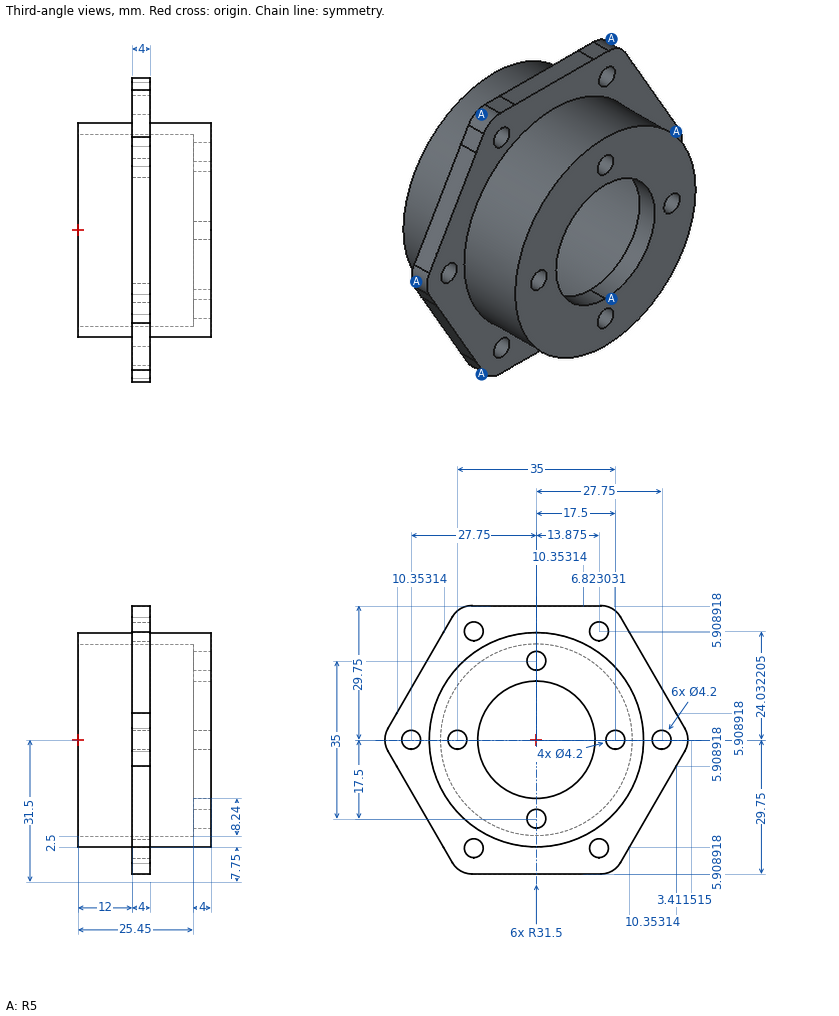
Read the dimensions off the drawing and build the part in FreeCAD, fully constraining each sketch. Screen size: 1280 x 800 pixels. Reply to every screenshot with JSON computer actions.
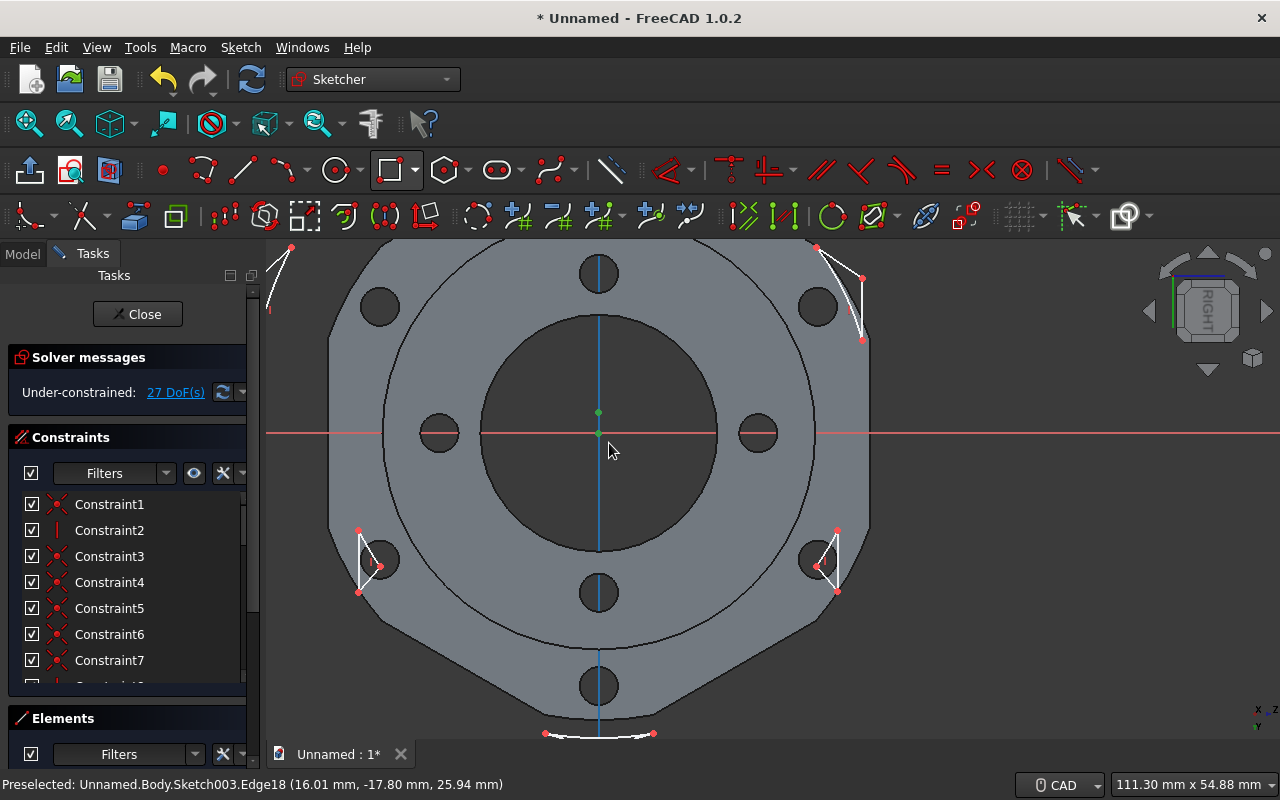
{"action": "key", "text": "c"}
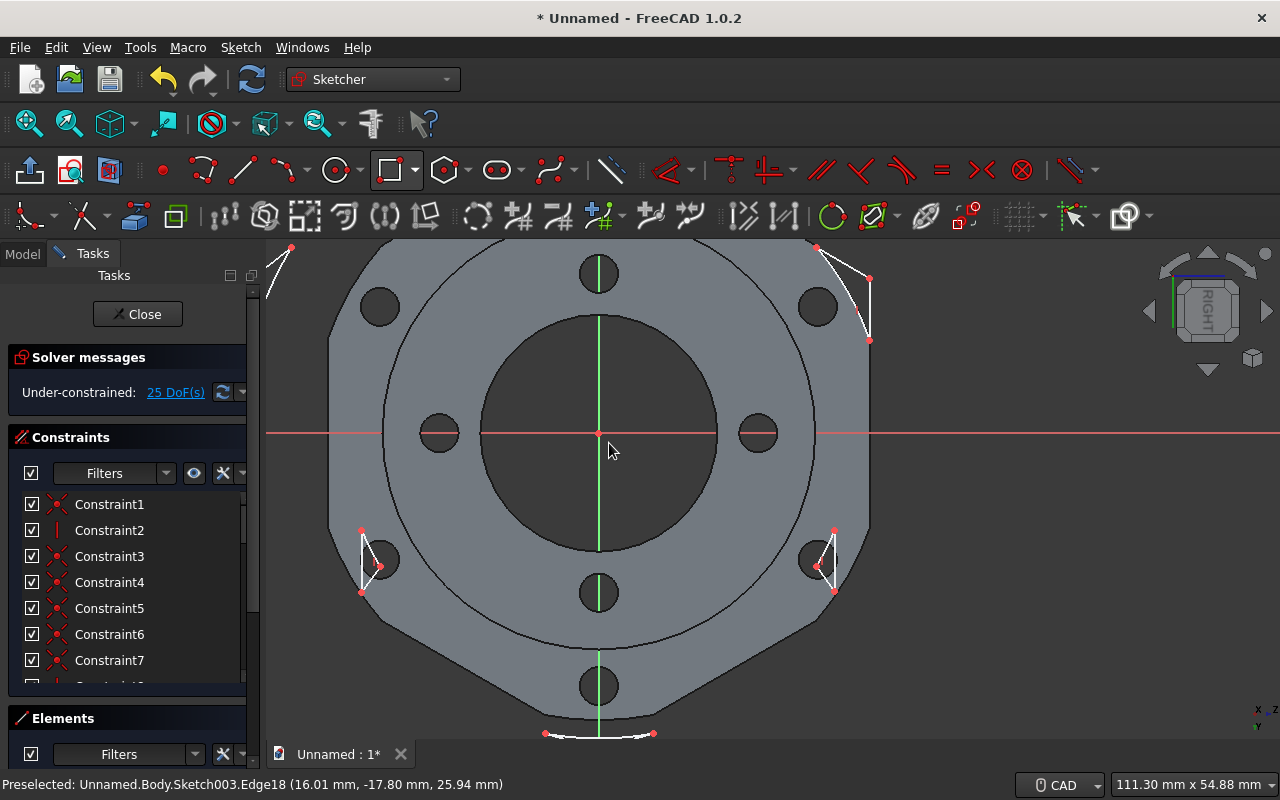
{"action": "left_click", "coordinate": [826, 548]}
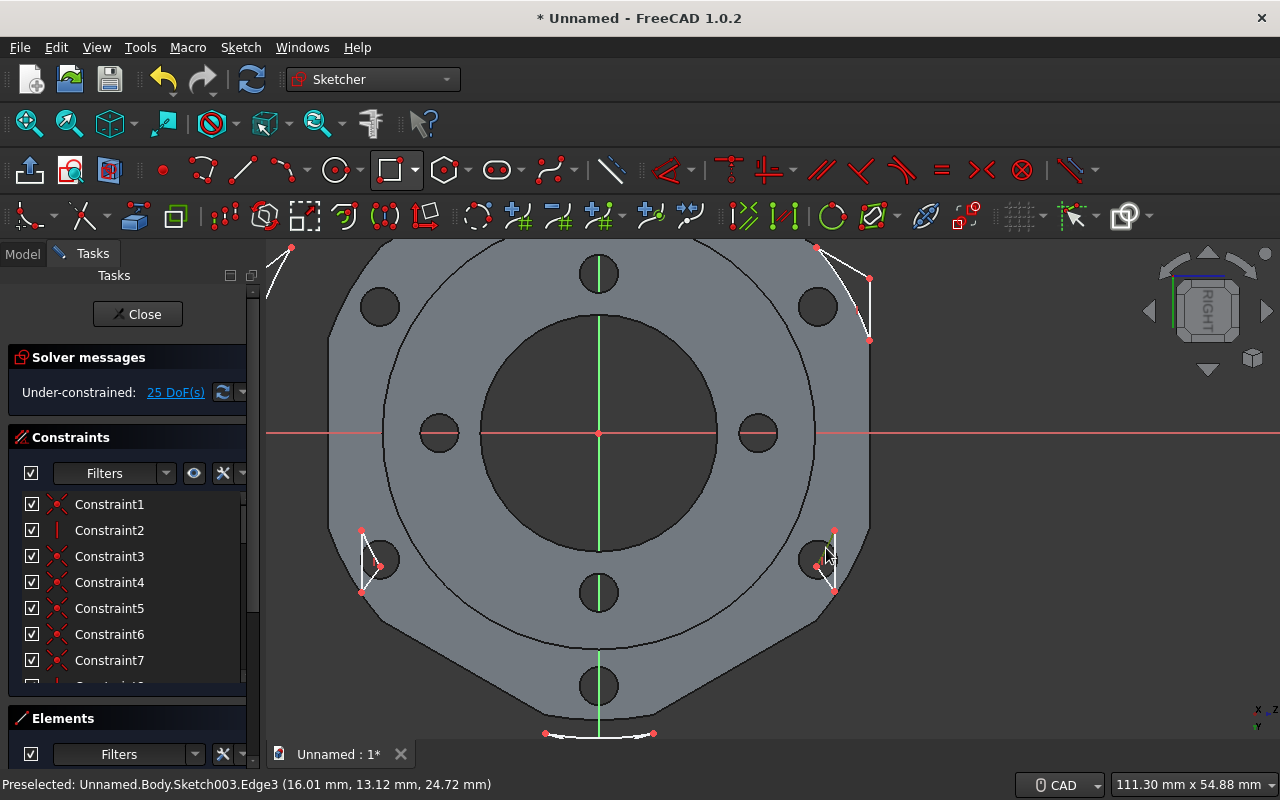
{"action": "scroll", "coordinate": [833, 557], "scroll_direction": "down", "scroll_amount": 3}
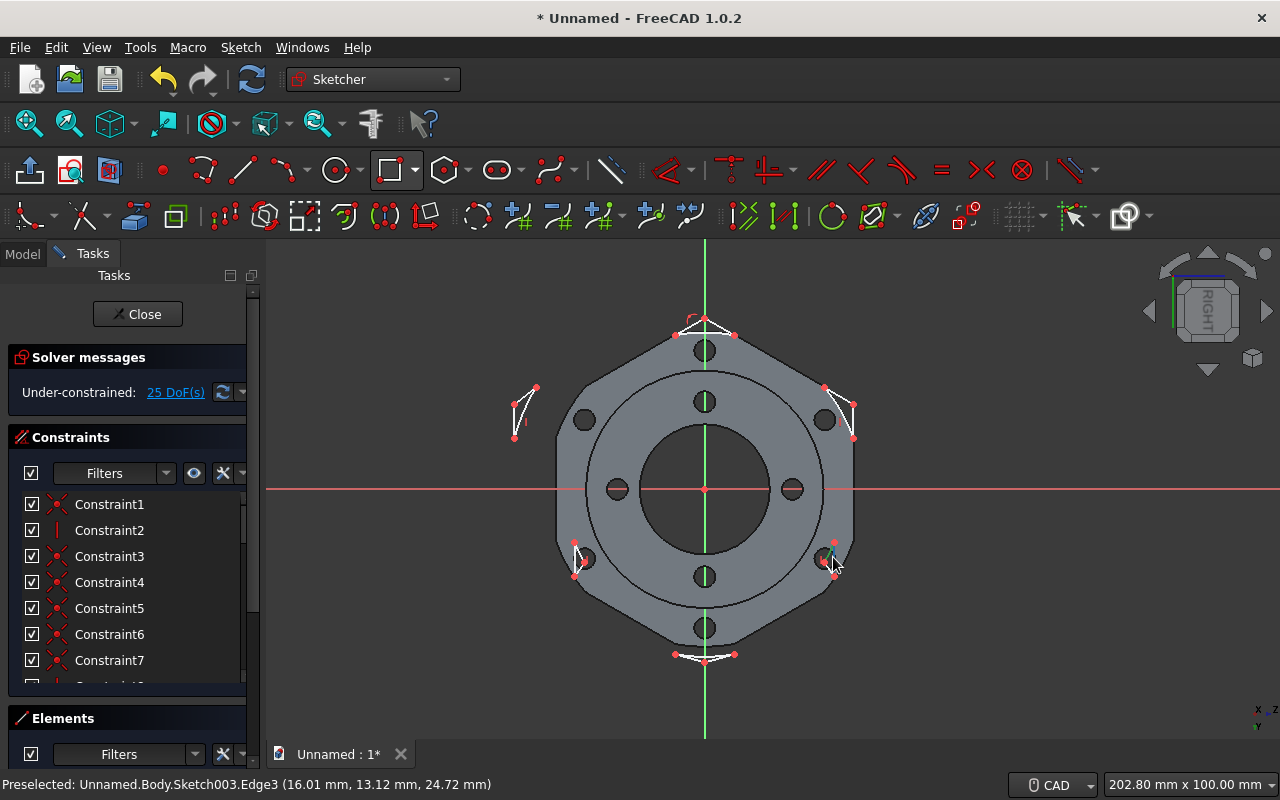
{"action": "scroll", "coordinate": [705, 657], "scroll_direction": "up", "scroll_amount": 5}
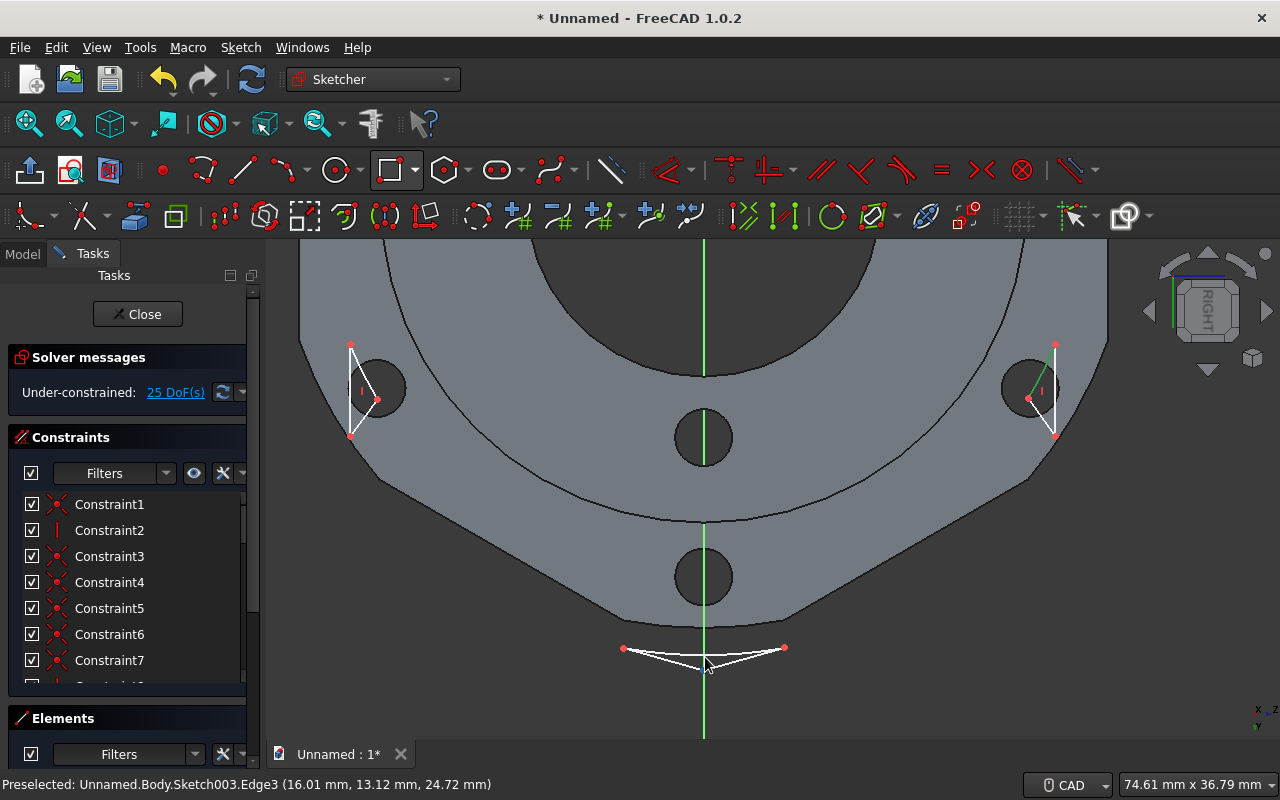
{"action": "left_click", "coordinate": [704, 655]}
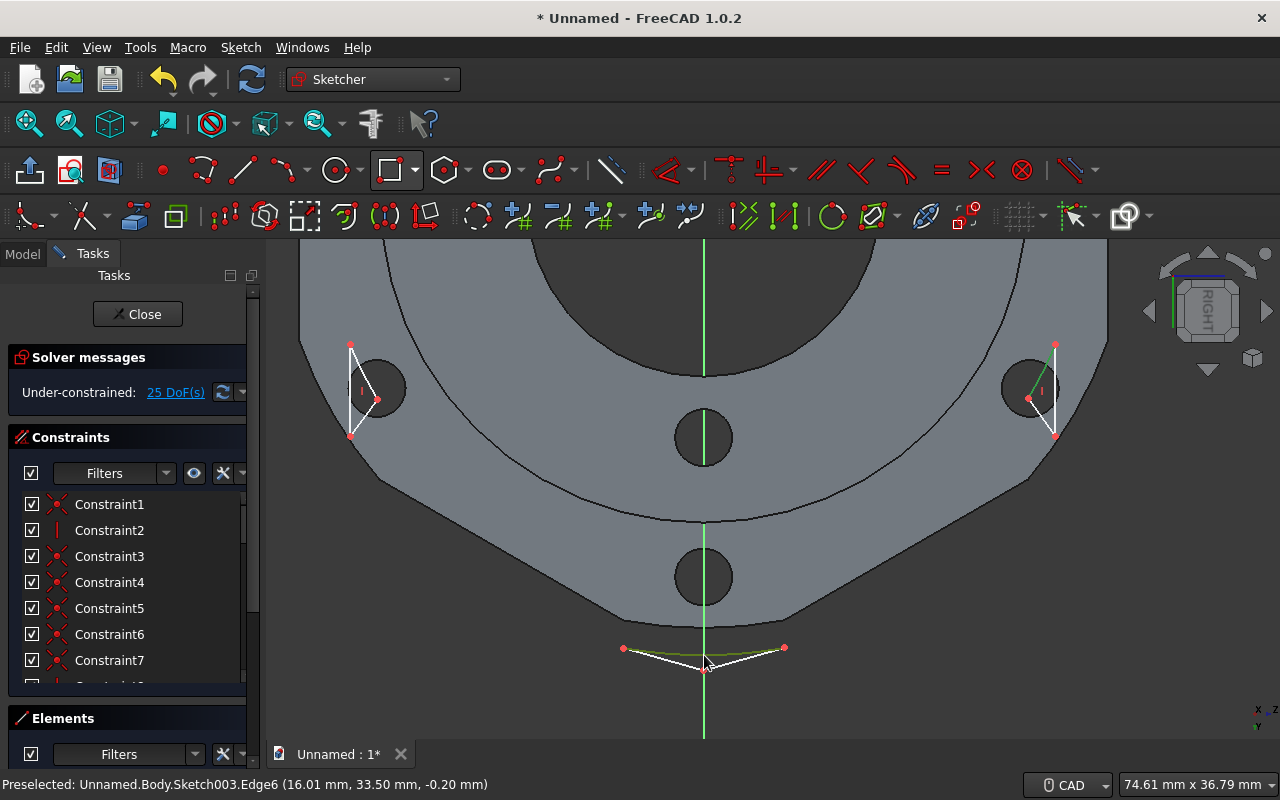
{"action": "left_click", "coordinate": [369, 383]}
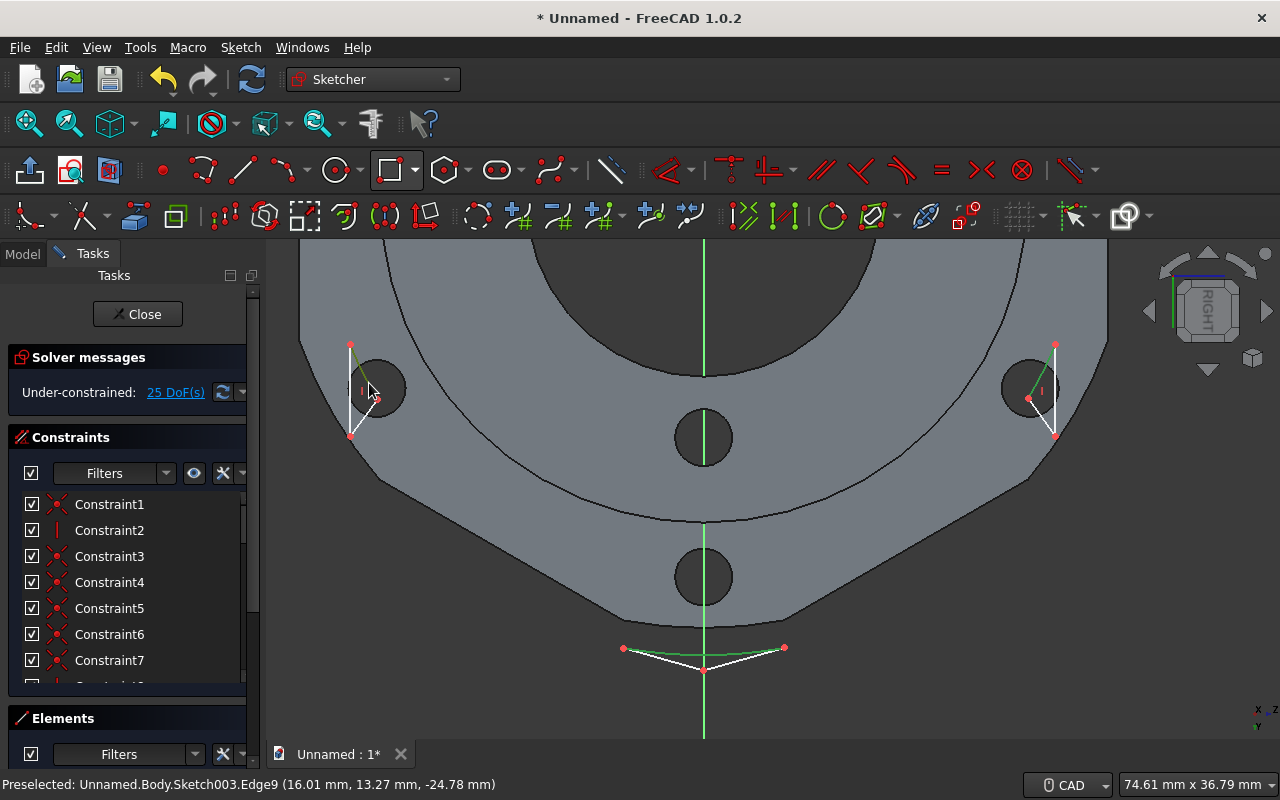
{"action": "scroll", "coordinate": [705, 657], "scroll_direction": "down", "scroll_amount": 5}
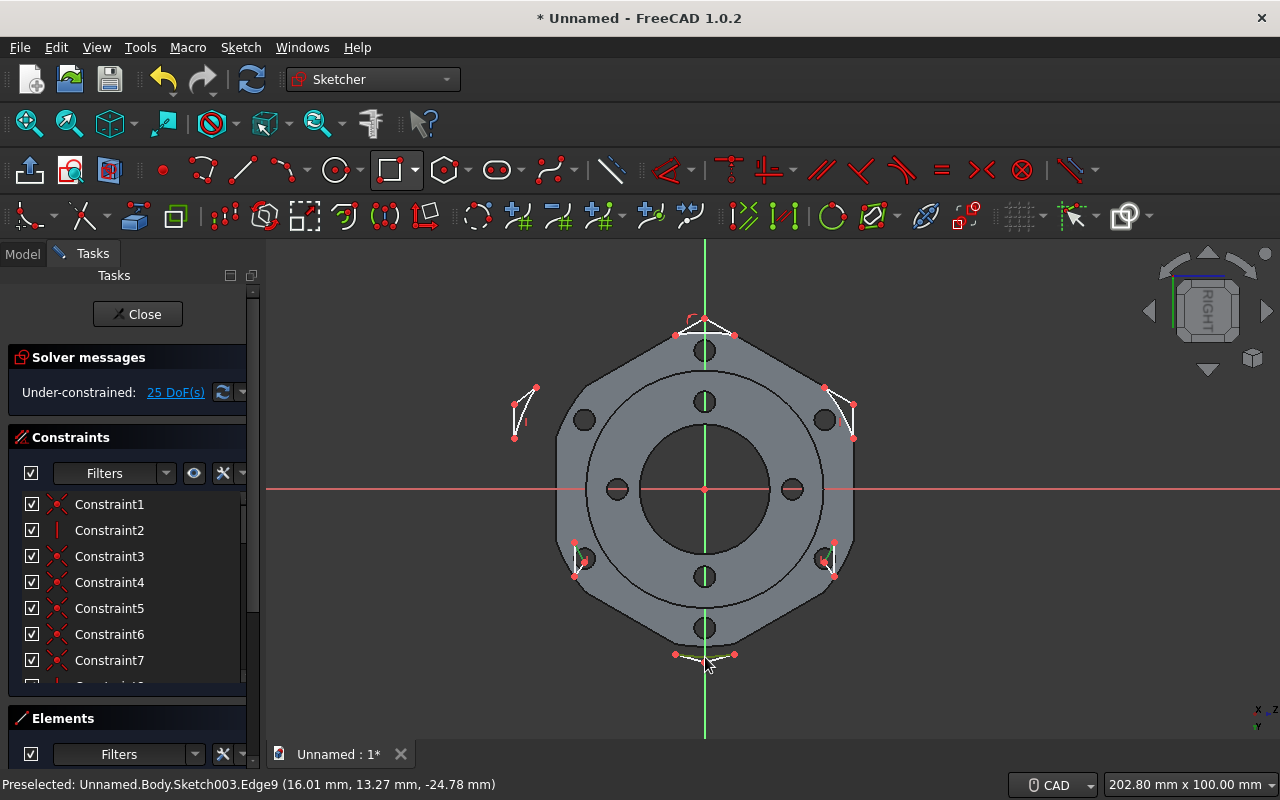
{"action": "scroll", "coordinate": [528, 402], "scroll_direction": "up", "scroll_amount": 4}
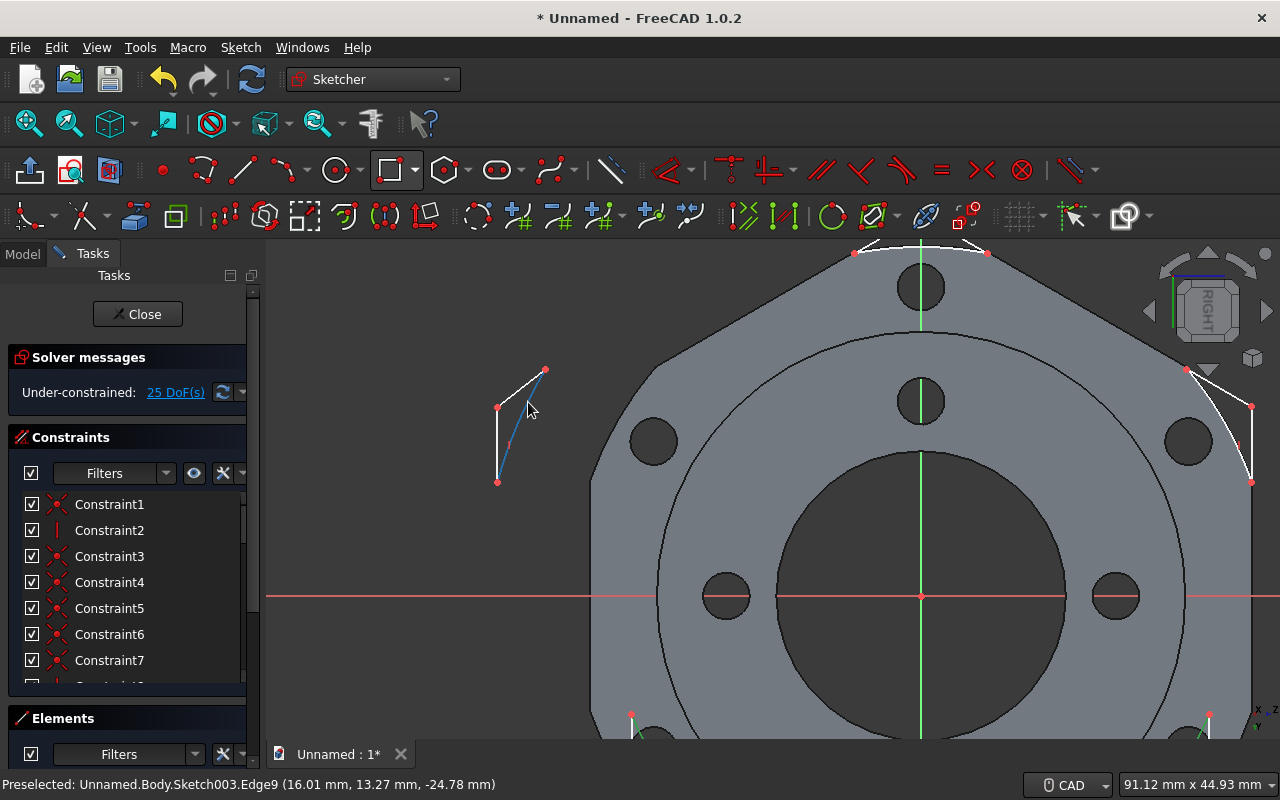
{"action": "left_click", "coordinate": [528, 402]}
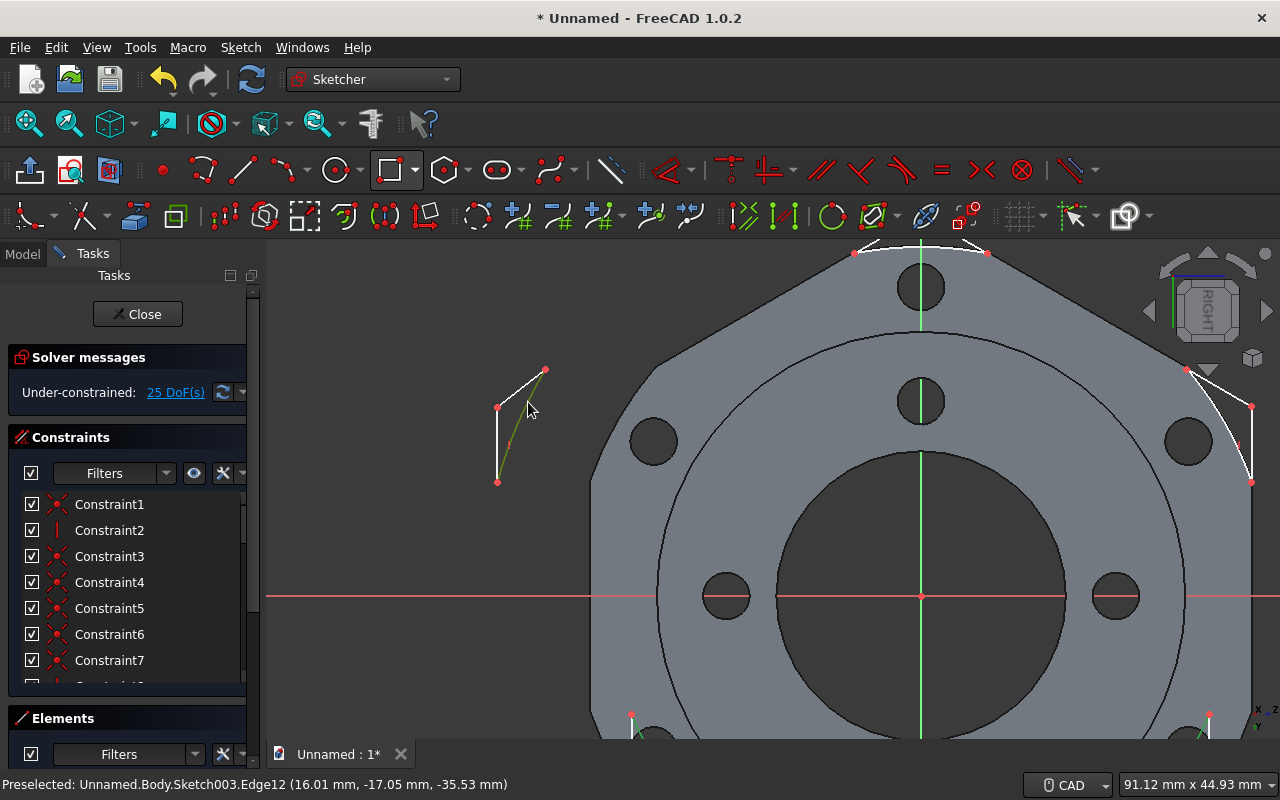
{"action": "scroll", "coordinate": [528, 402], "scroll_direction": "down", "scroll_amount": 4}